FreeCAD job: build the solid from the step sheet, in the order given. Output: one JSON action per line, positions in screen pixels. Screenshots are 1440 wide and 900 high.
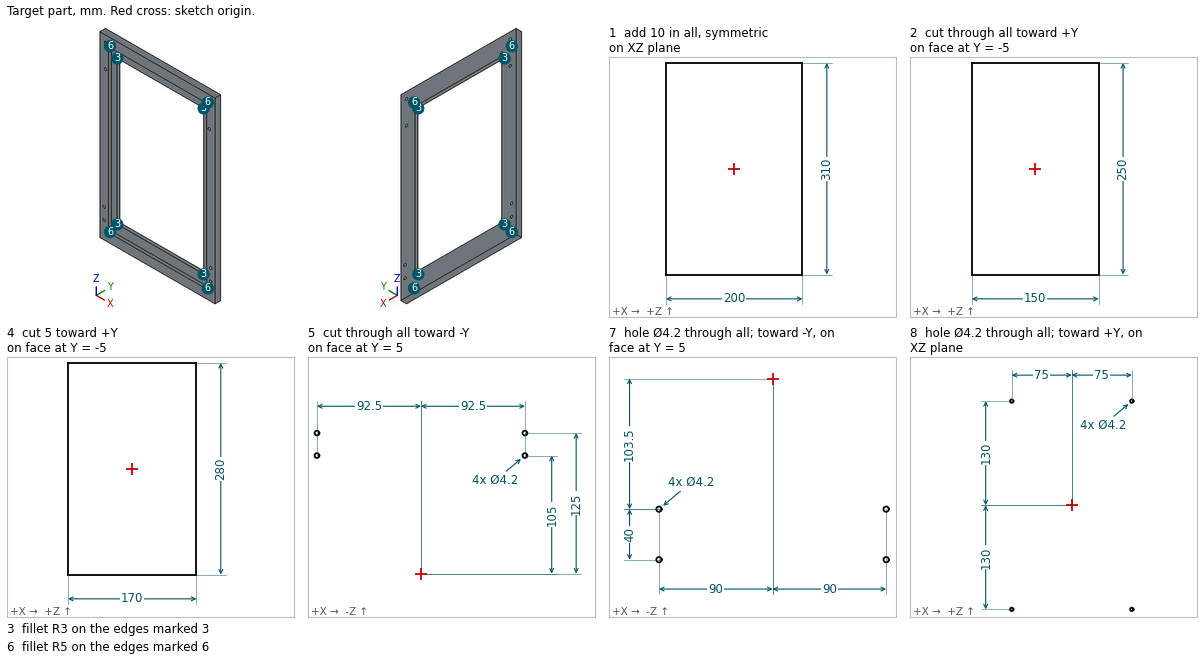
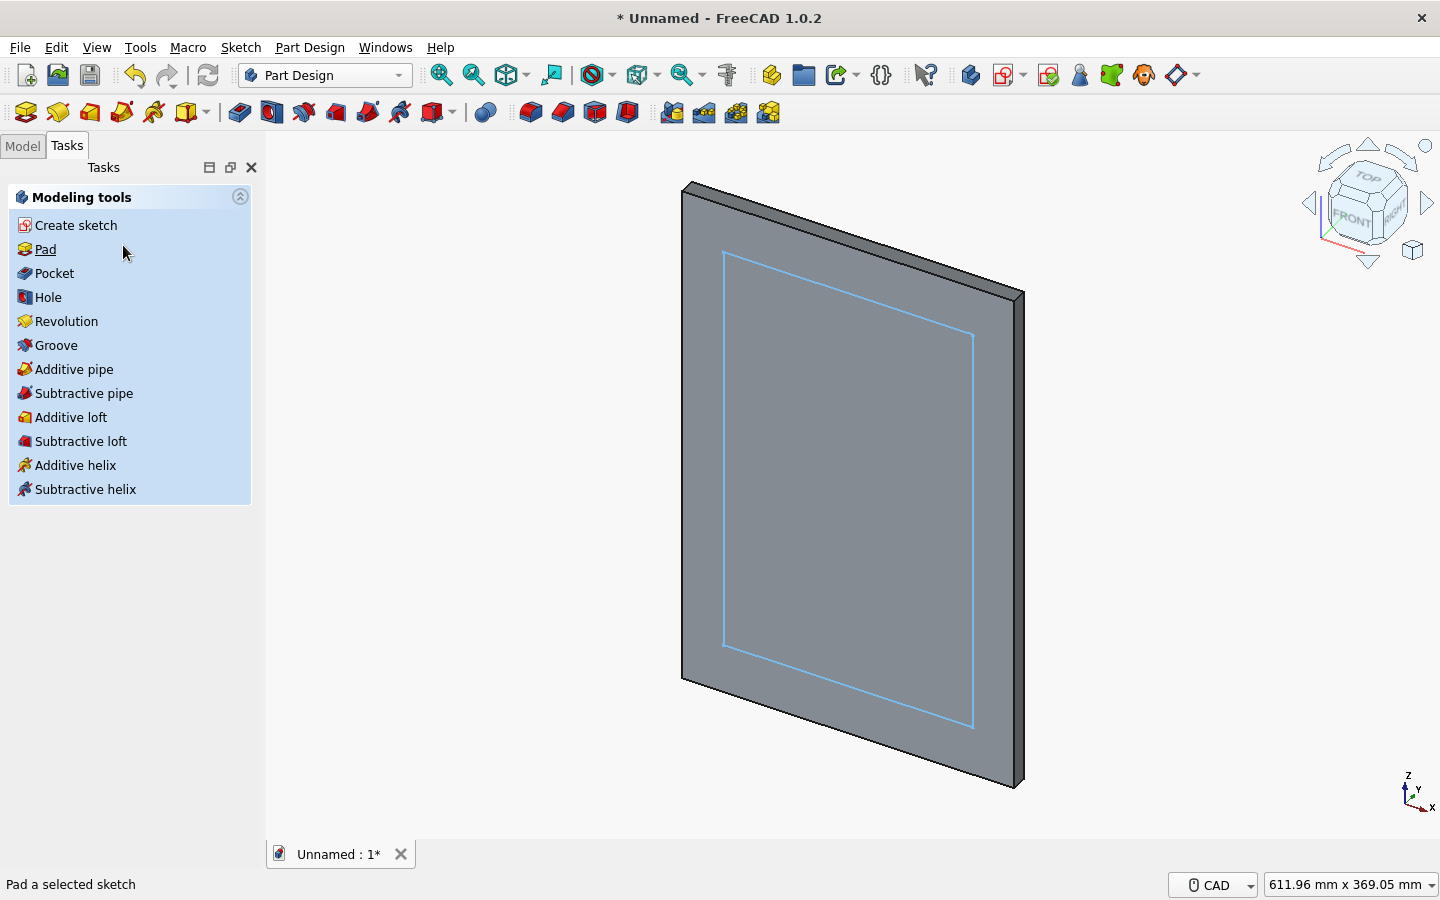
{"action": "left_click", "coordinate": [240, 112]}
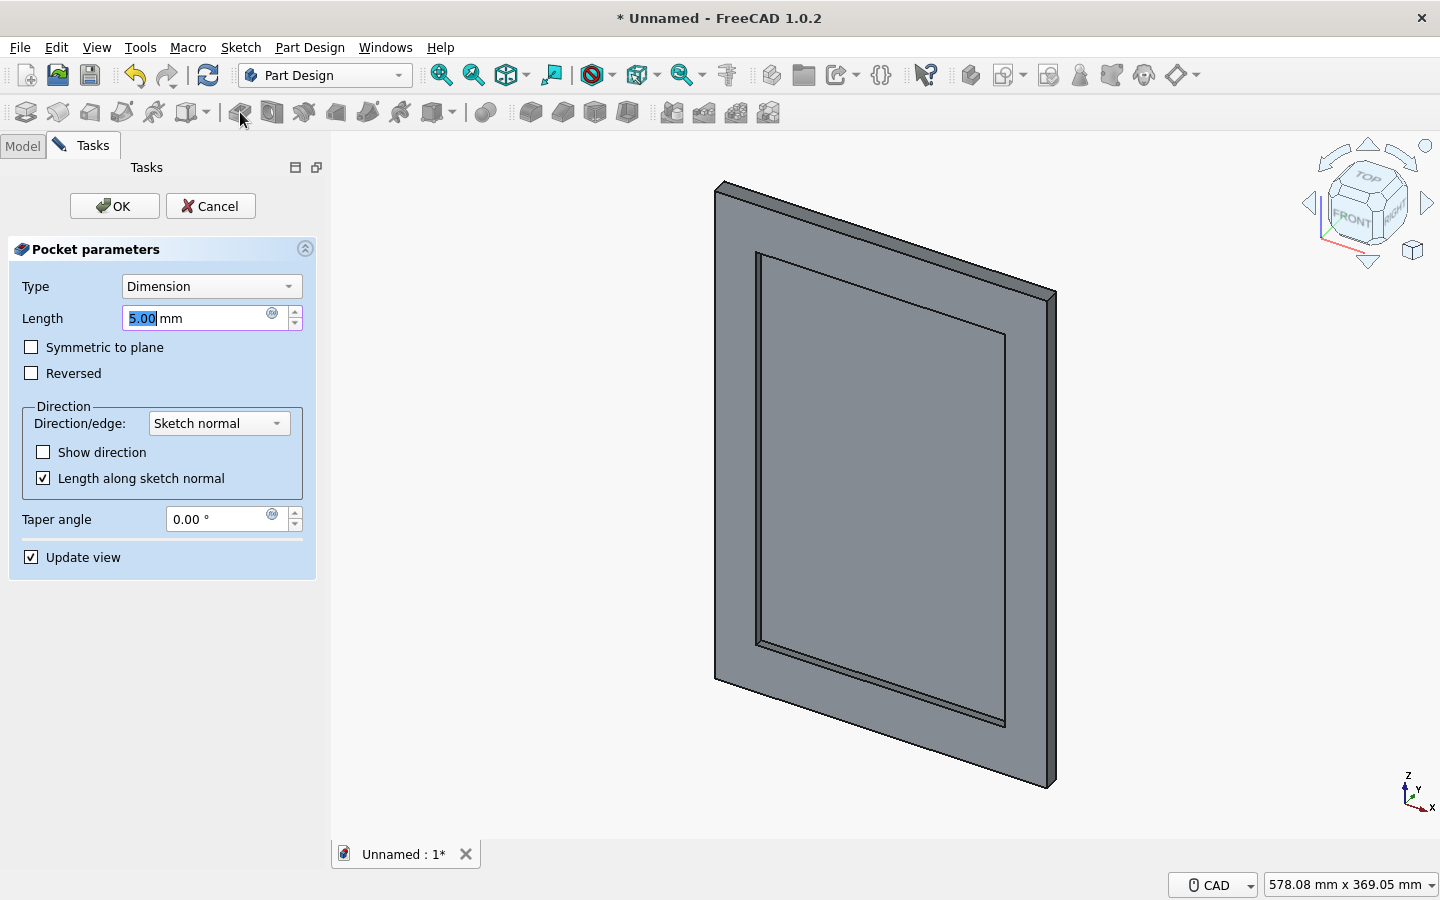
{"action": "left_click", "coordinate": [212, 286]}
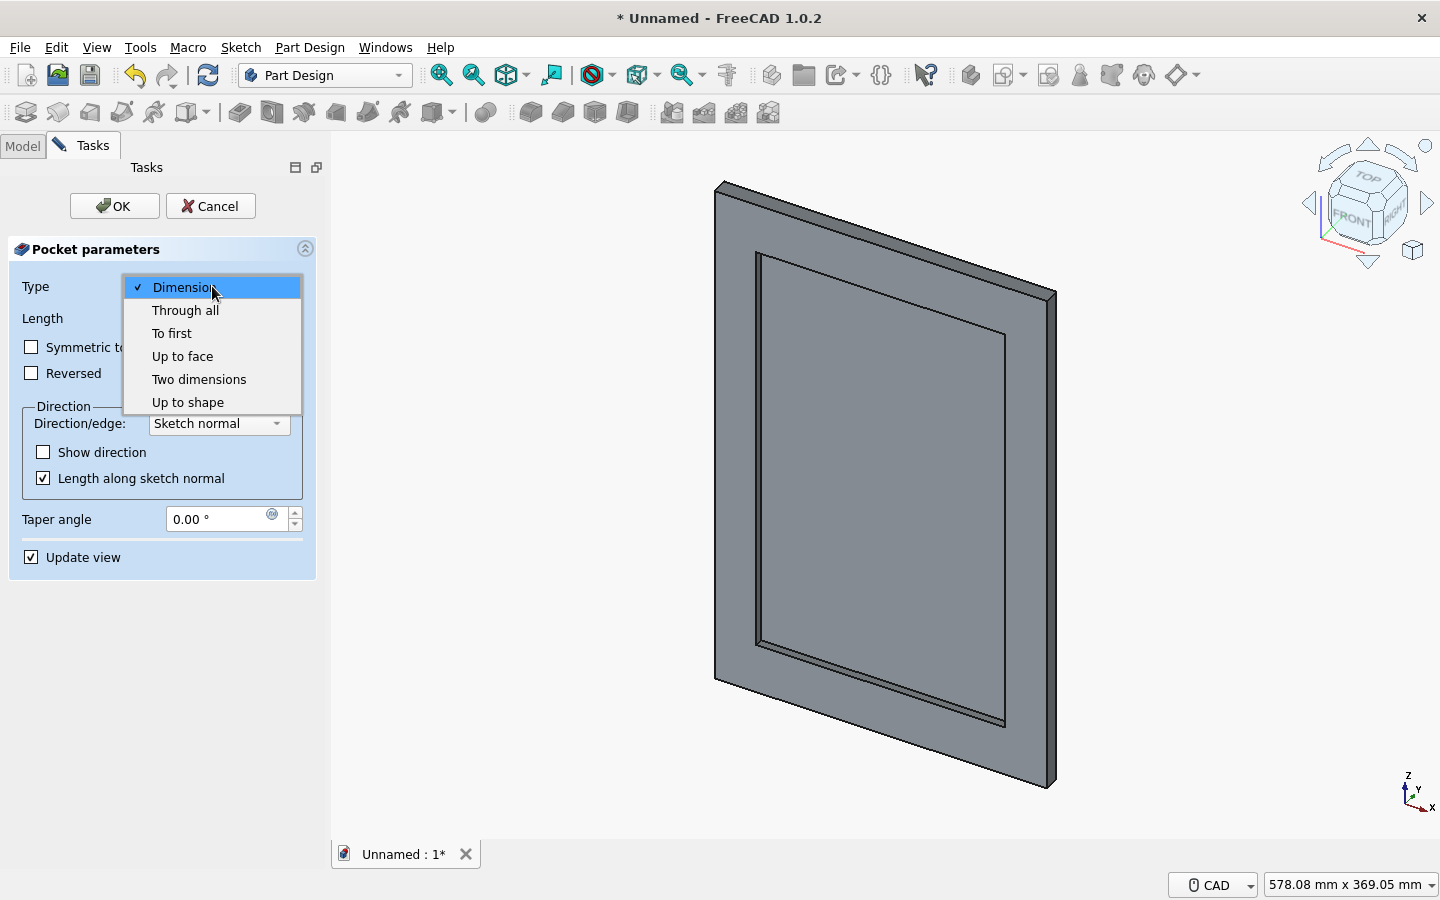
{"action": "left_click", "coordinate": [212, 310]}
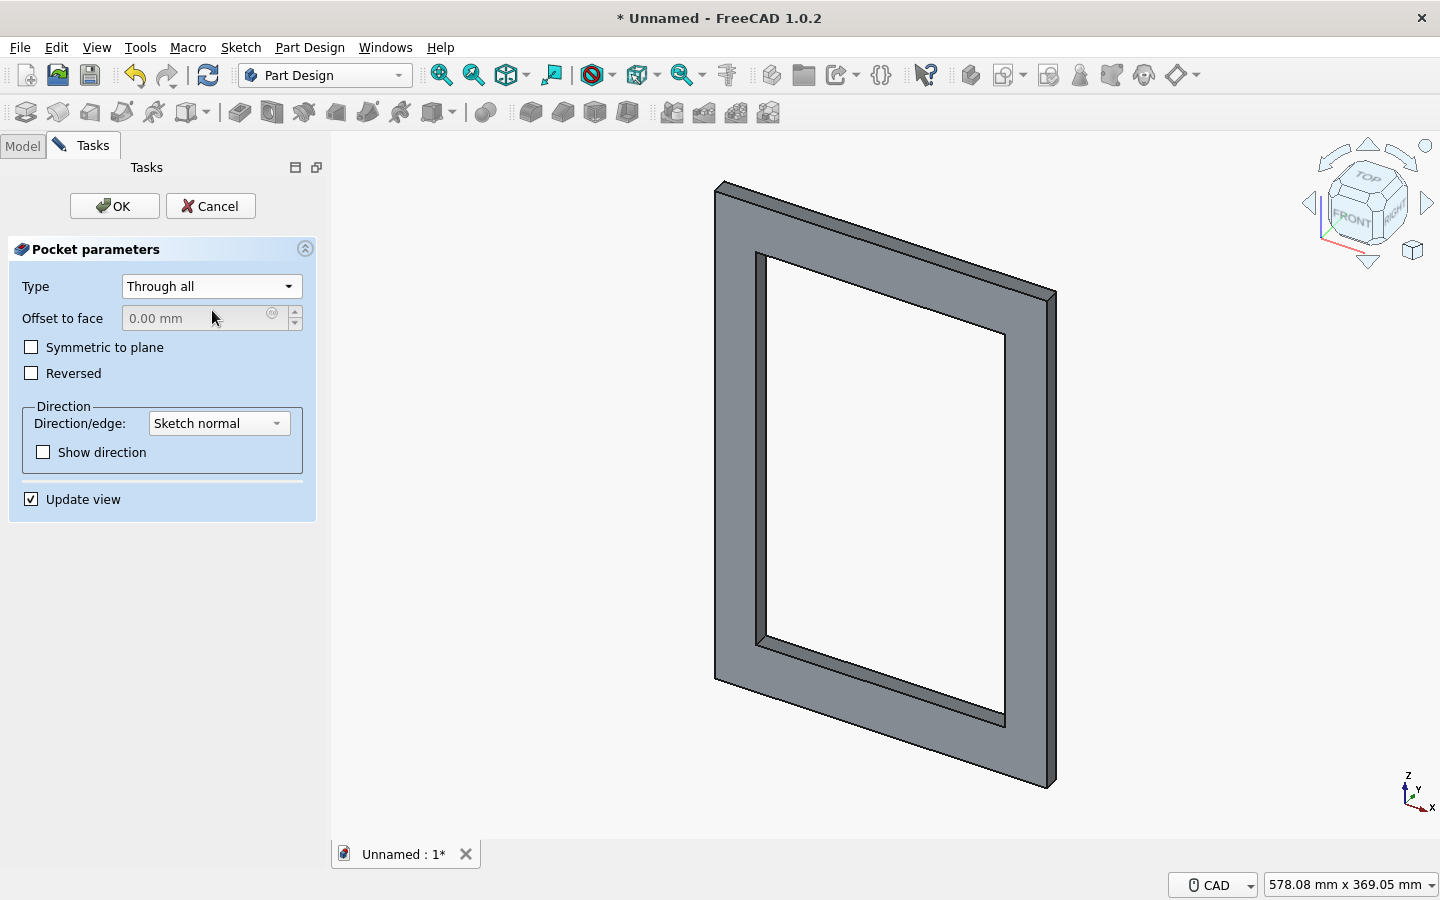
{"action": "left_click", "coordinate": [115, 206]}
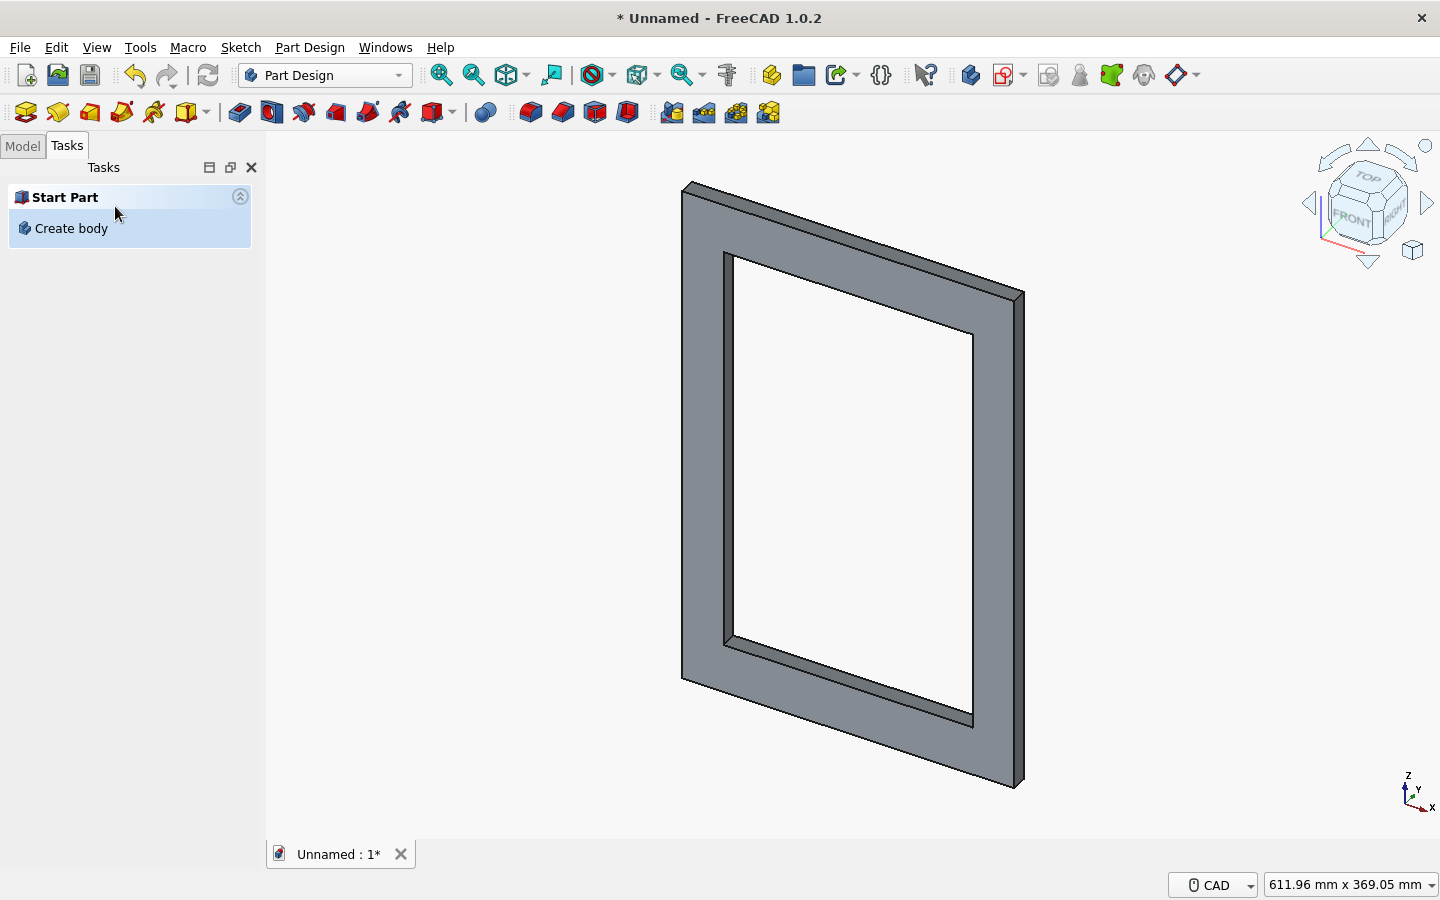
{"action": "scroll", "coordinate": [978, 329], "scroll_direction": "up", "scroll_amount": 4}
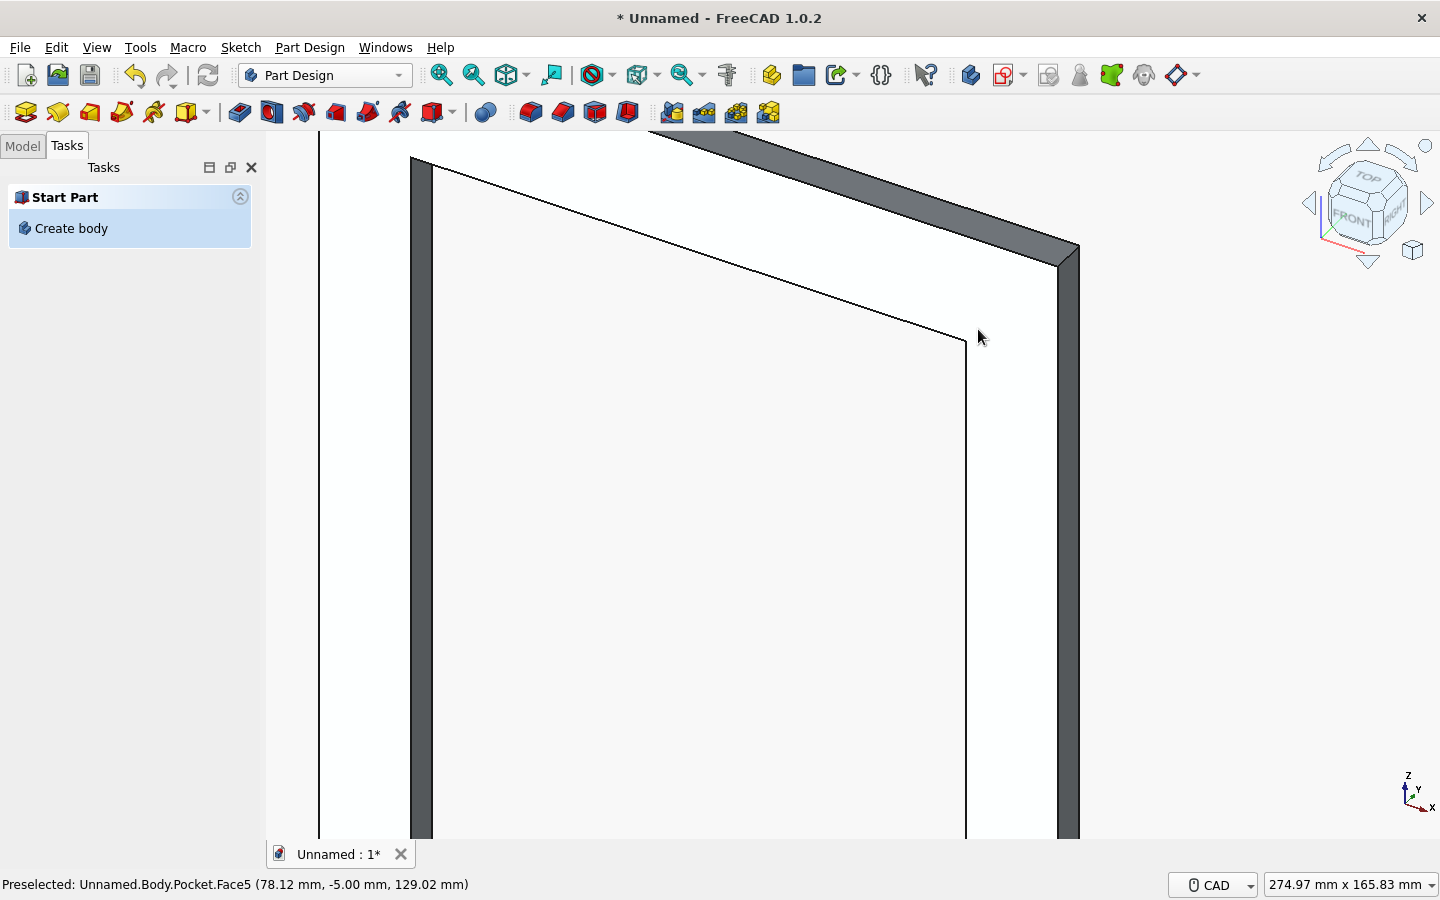
{"action": "left_click", "coordinate": [442, 76]}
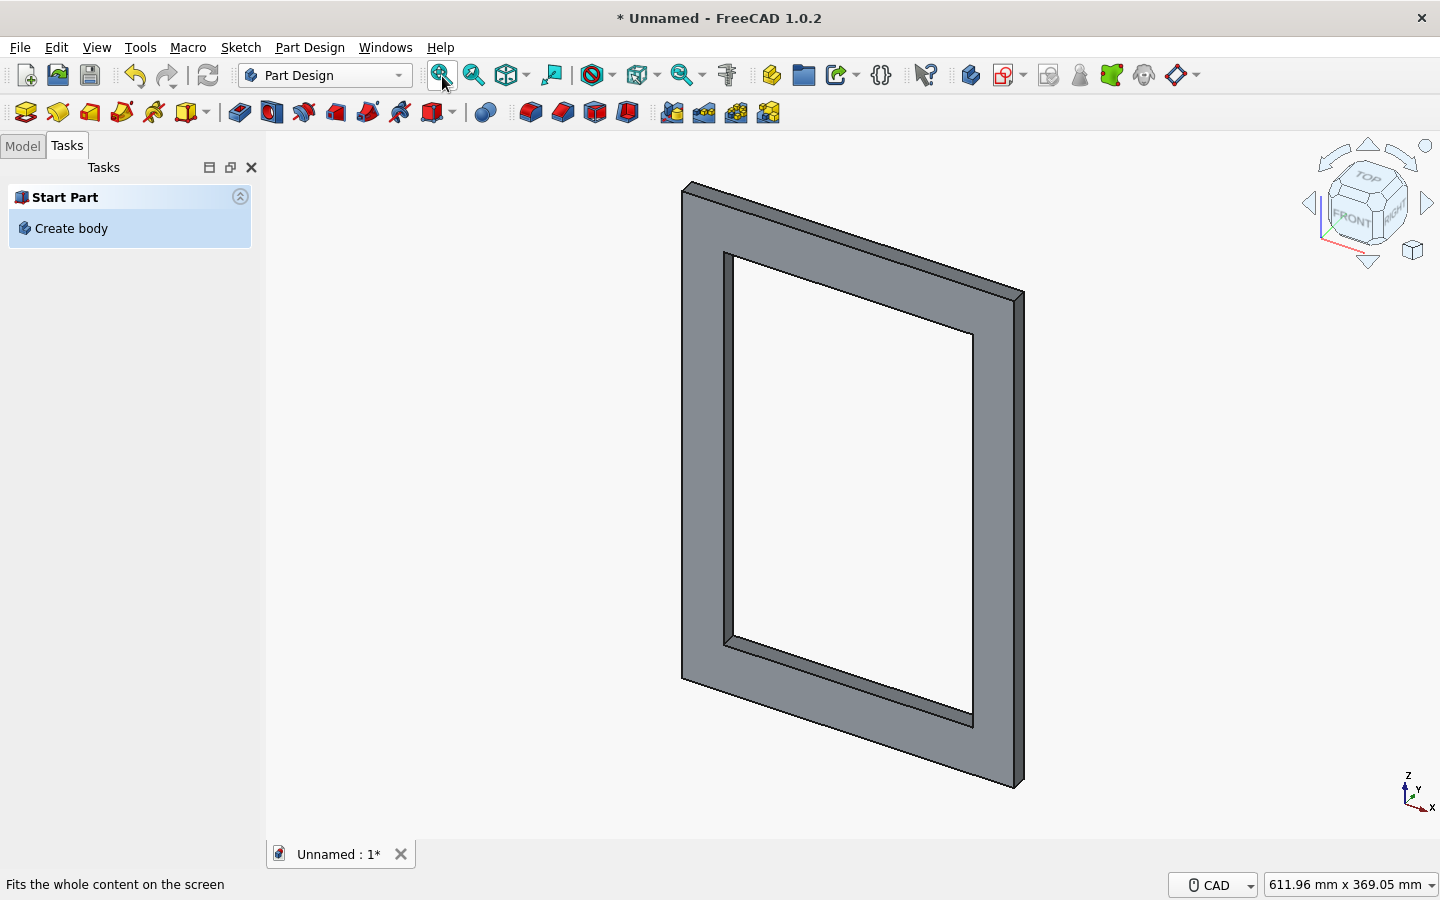
{"action": "key", "text": "0"}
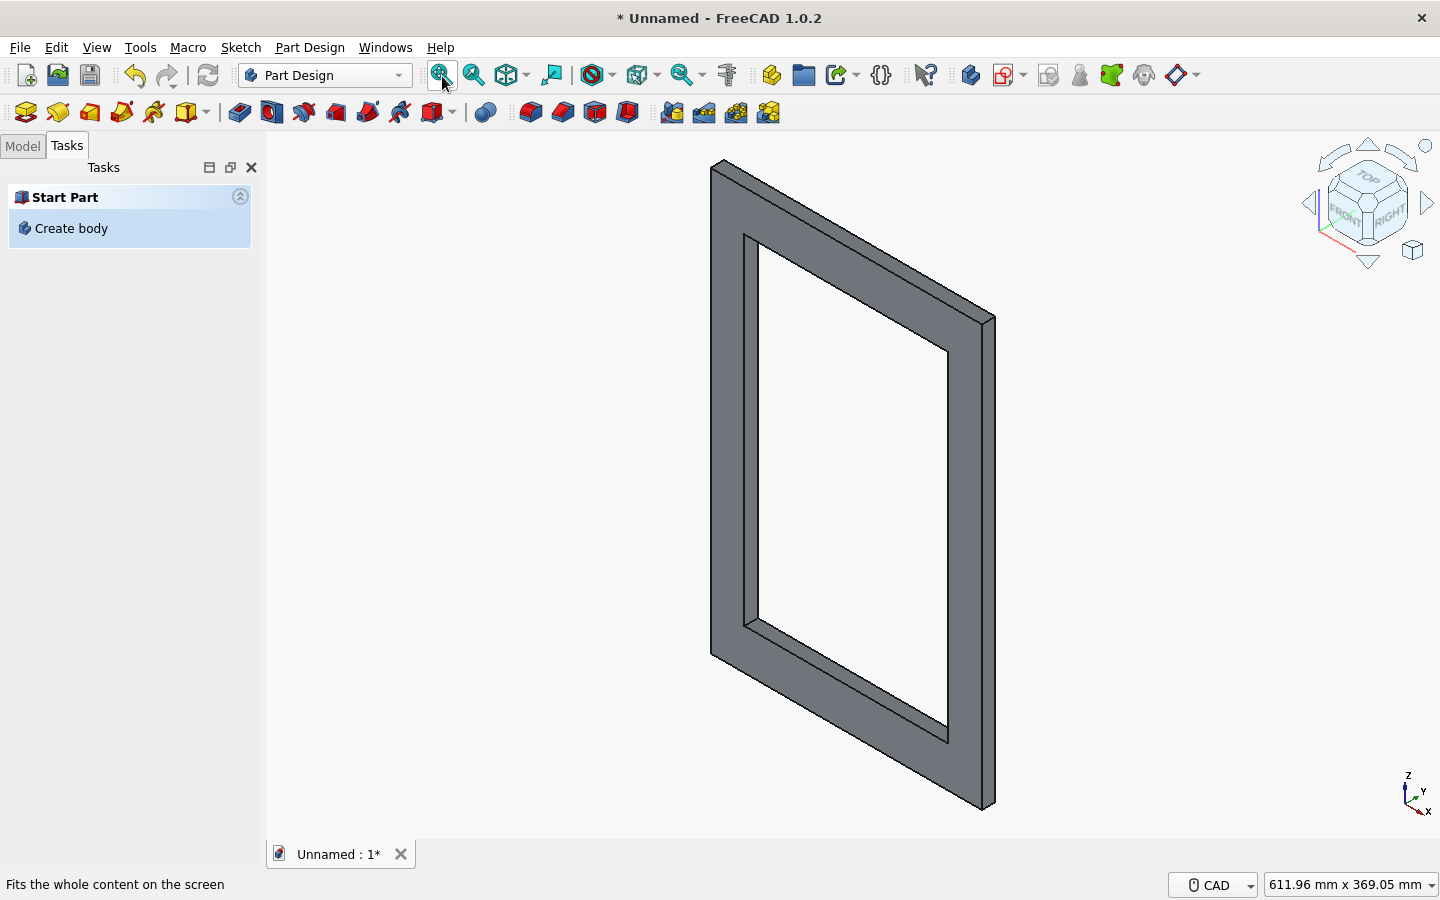
{"action": "scroll", "coordinate": [955, 347], "scroll_direction": "up", "scroll_amount": 4}